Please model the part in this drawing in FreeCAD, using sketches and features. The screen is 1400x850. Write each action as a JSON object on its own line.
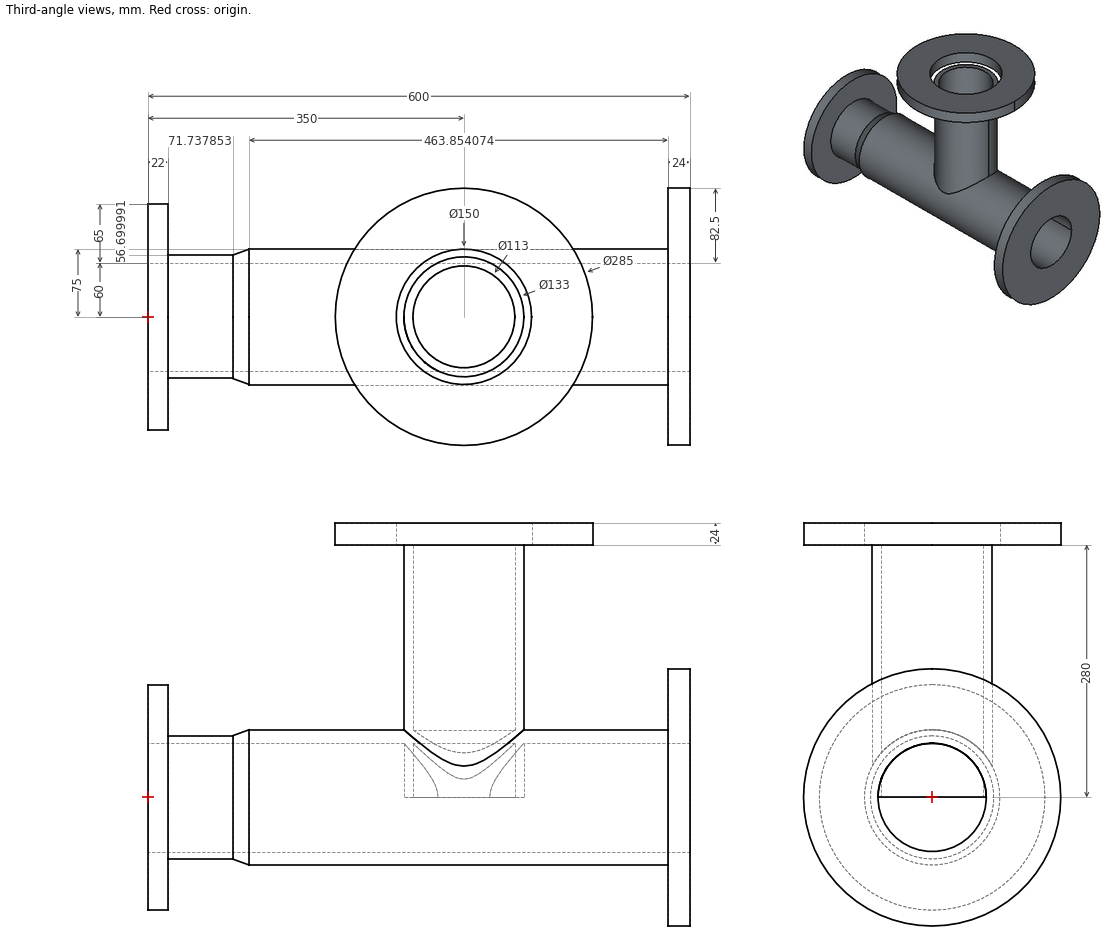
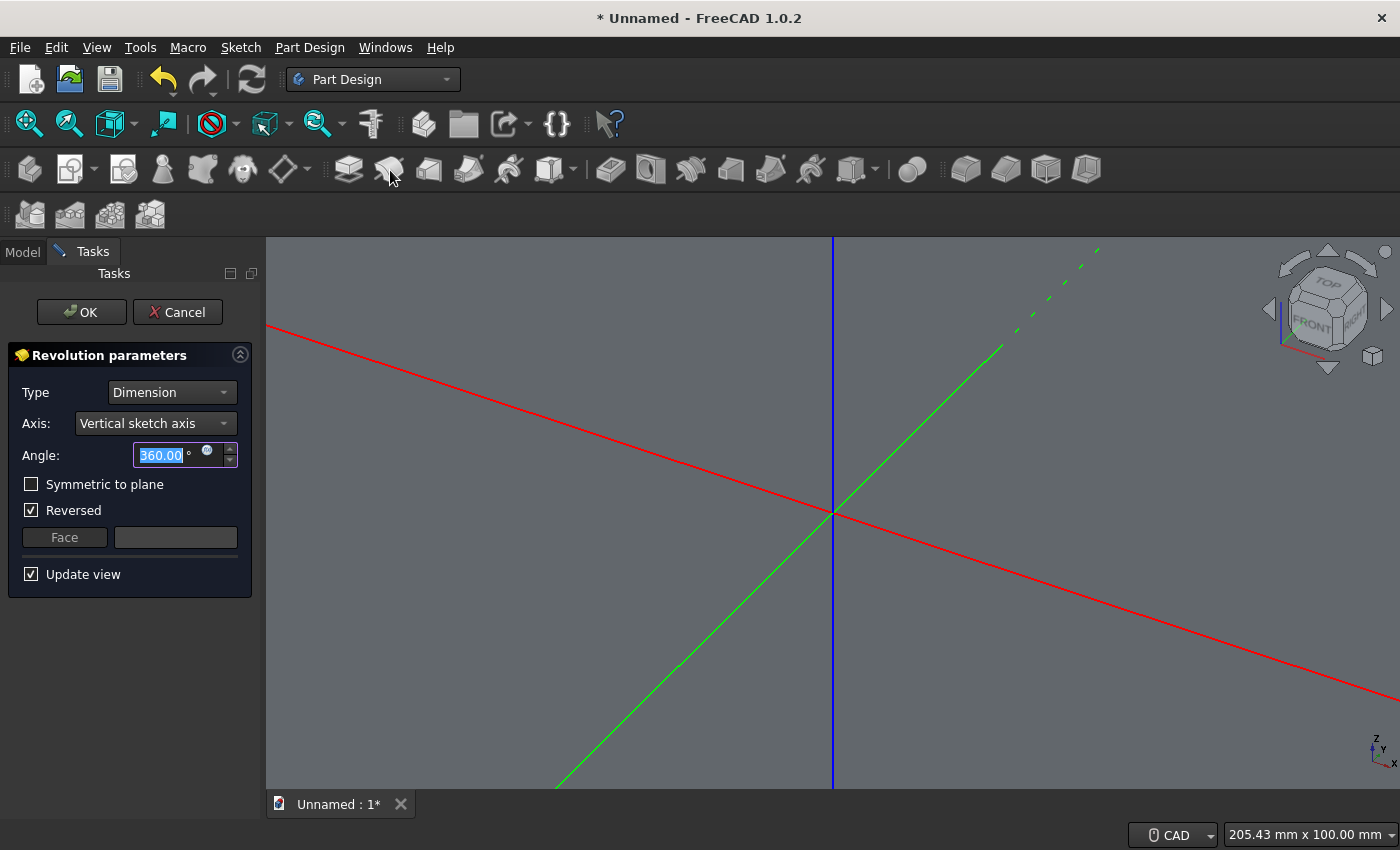
{"action": "left_click", "coordinate": [156, 424]}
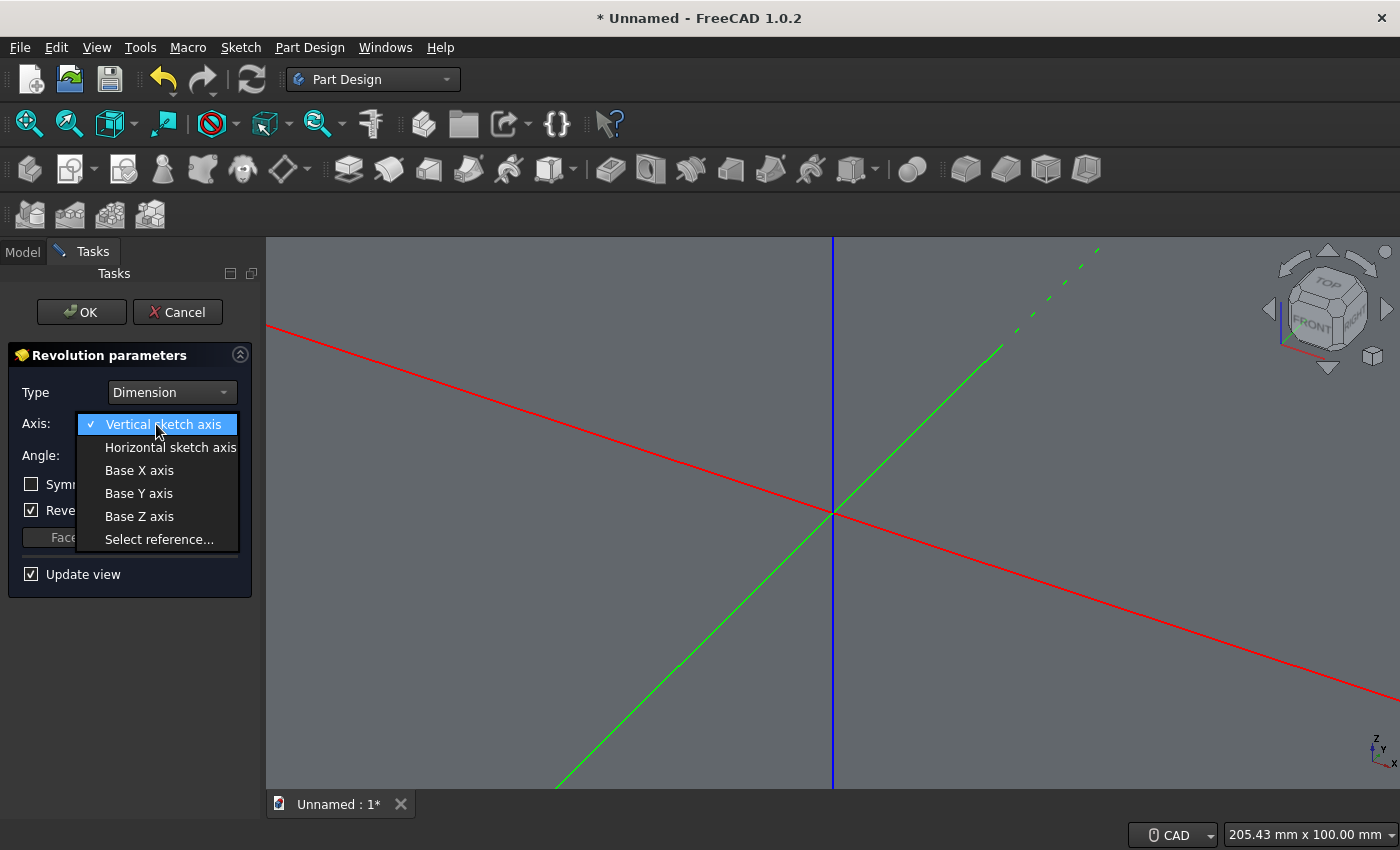
{"action": "left_click", "coordinate": [156, 448]}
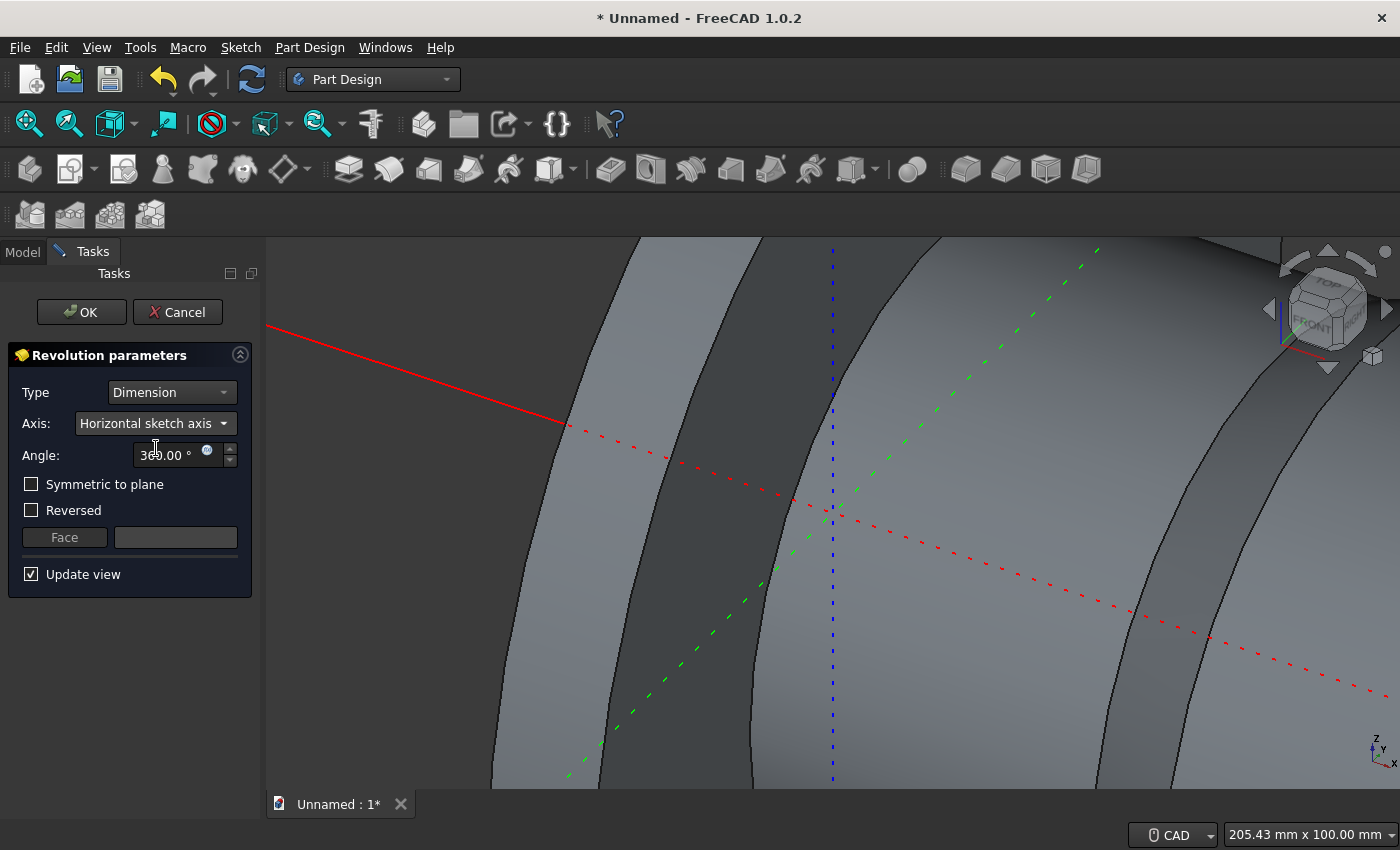
{"action": "left_click", "coordinate": [82, 312]}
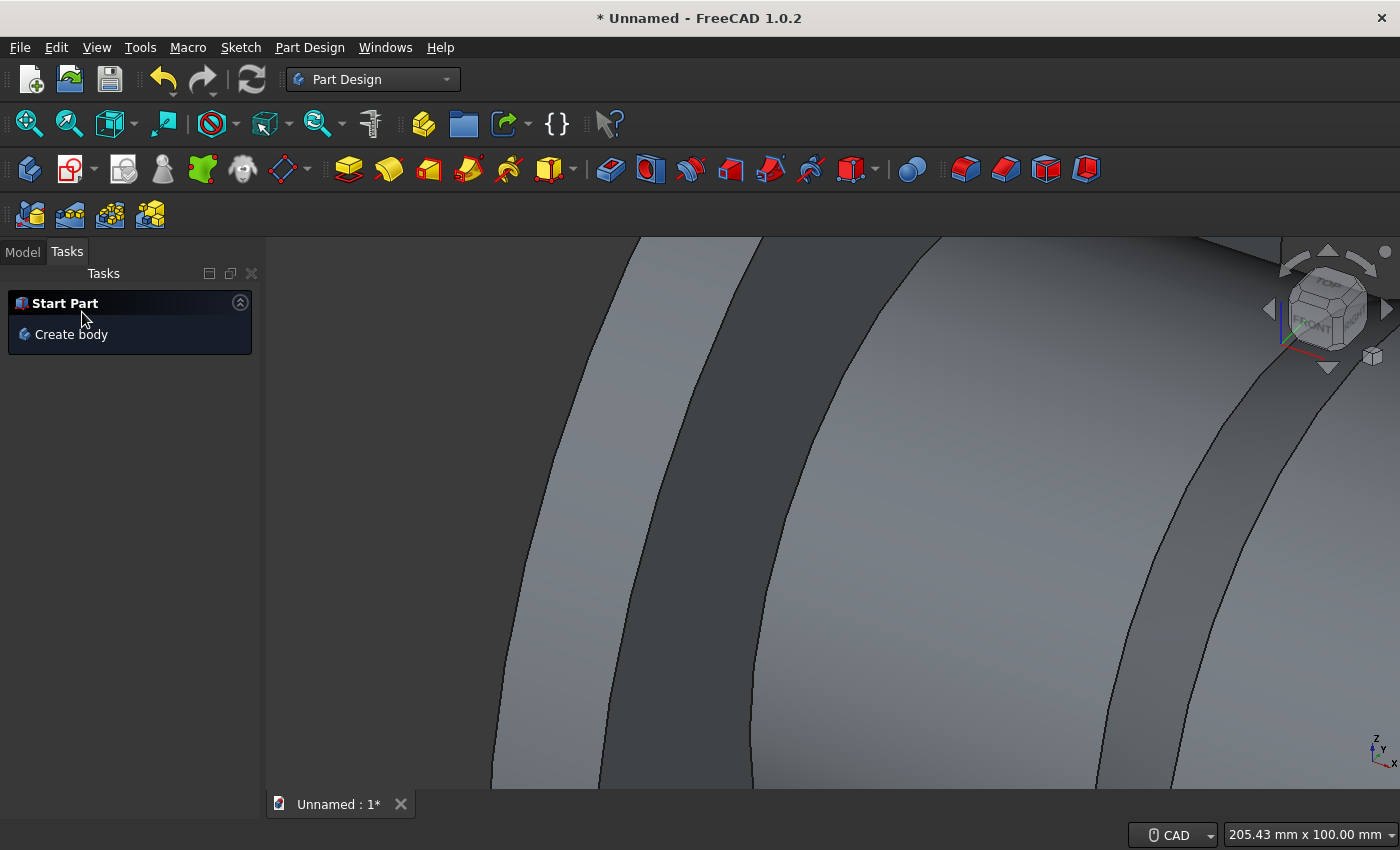
{"action": "key", "text": "v f"}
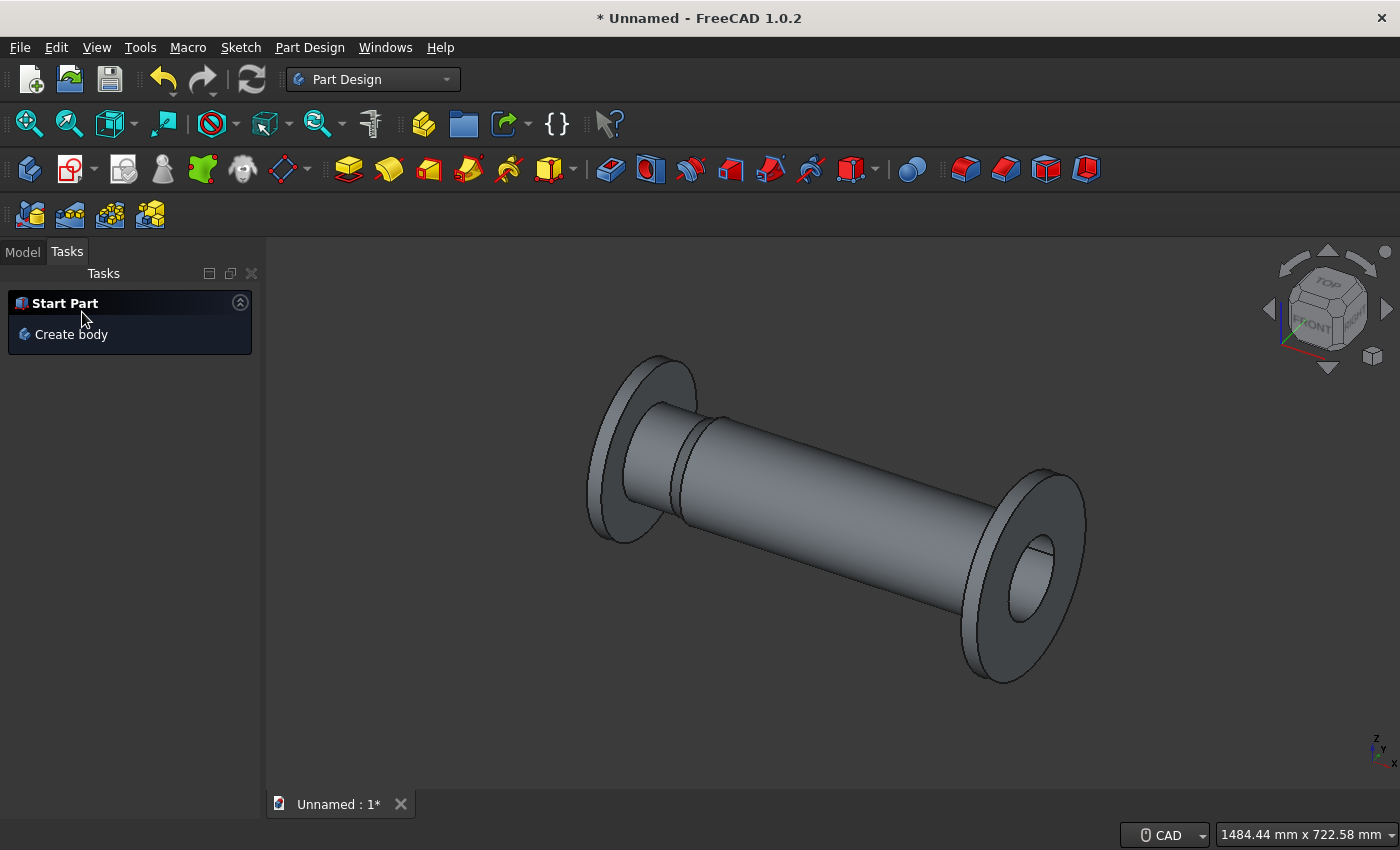
{"action": "left_click", "coordinate": [70, 170]}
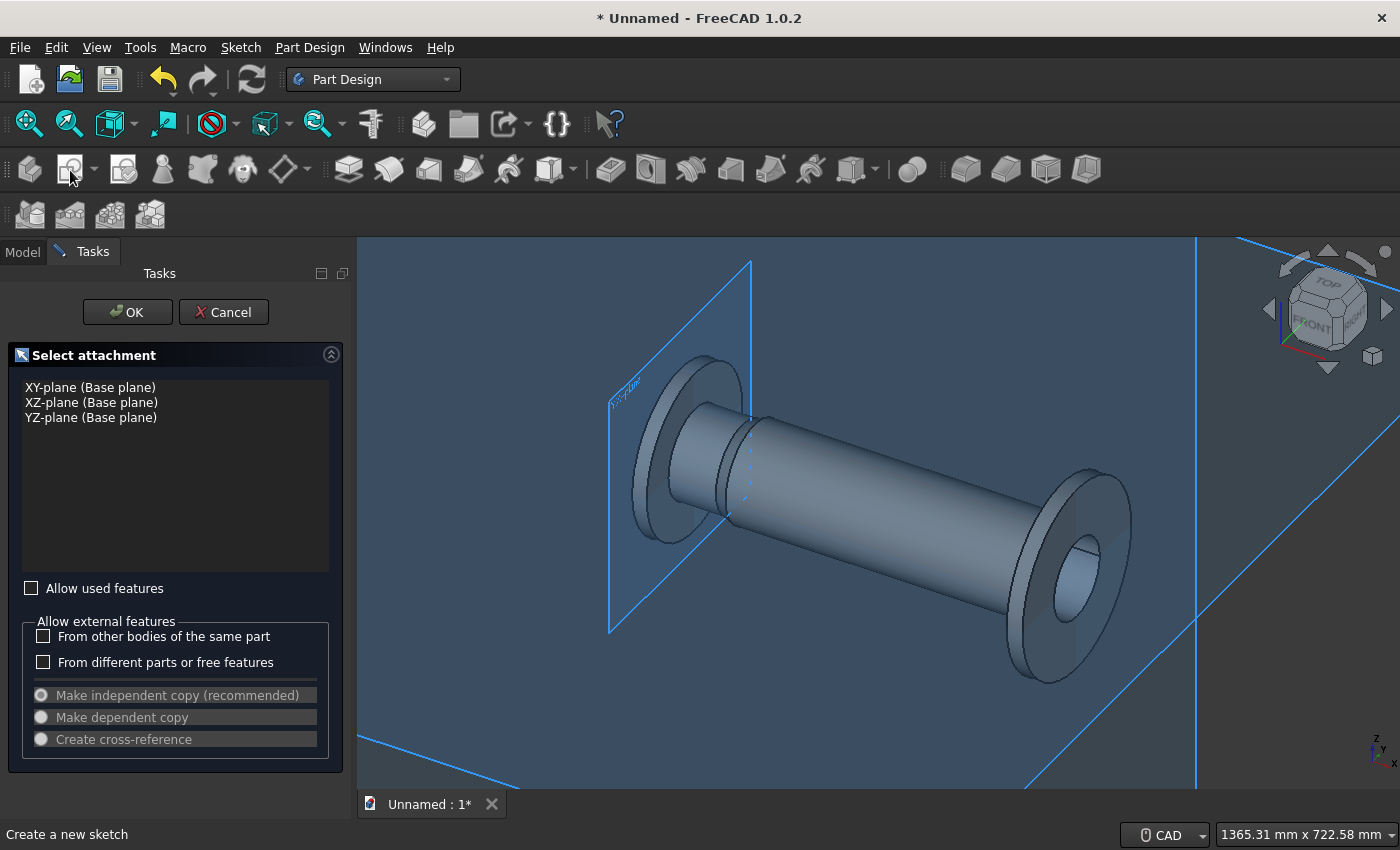
{"action": "left_click", "coordinate": [82, 388]}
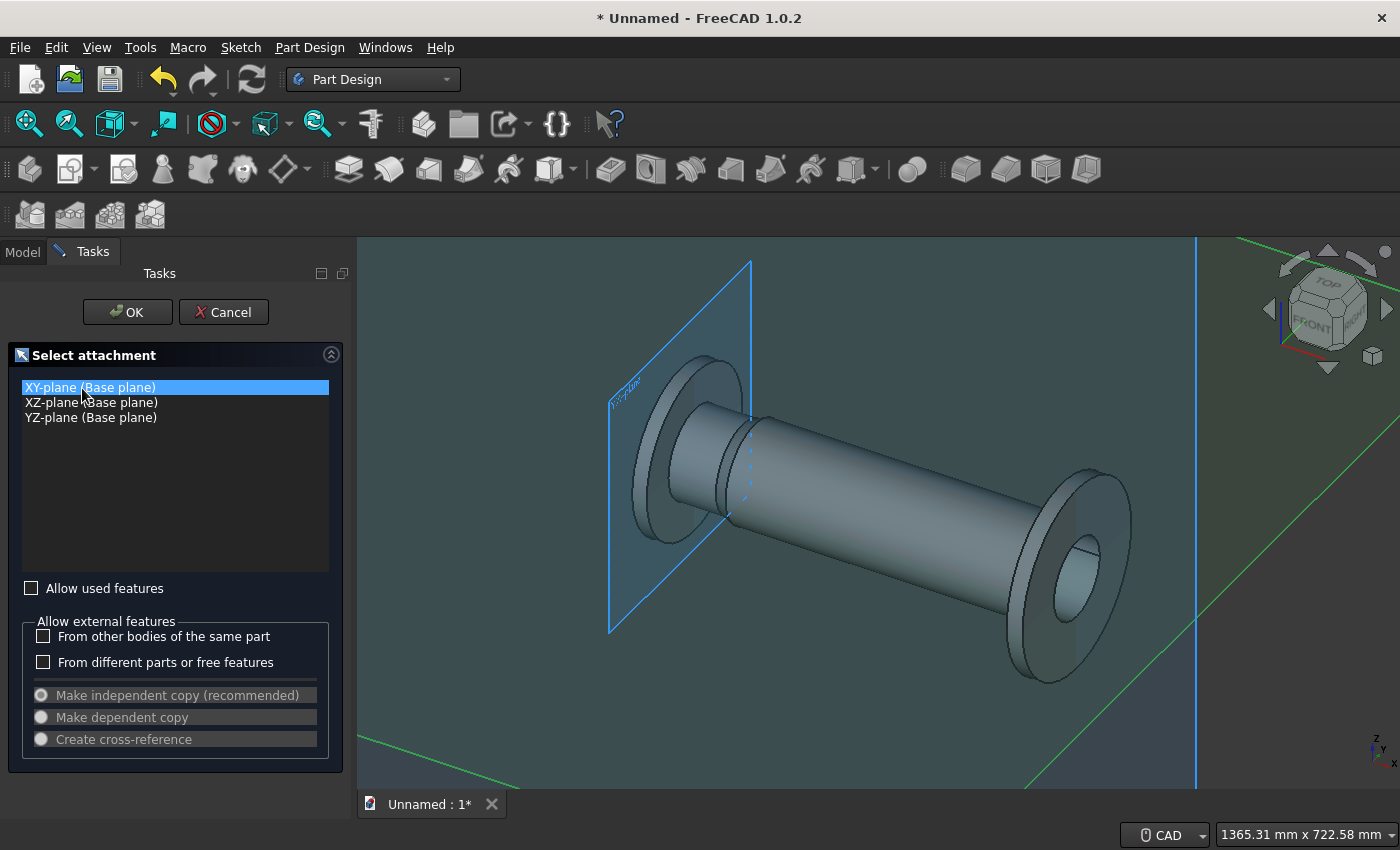
{"action": "left_click", "coordinate": [128, 312]}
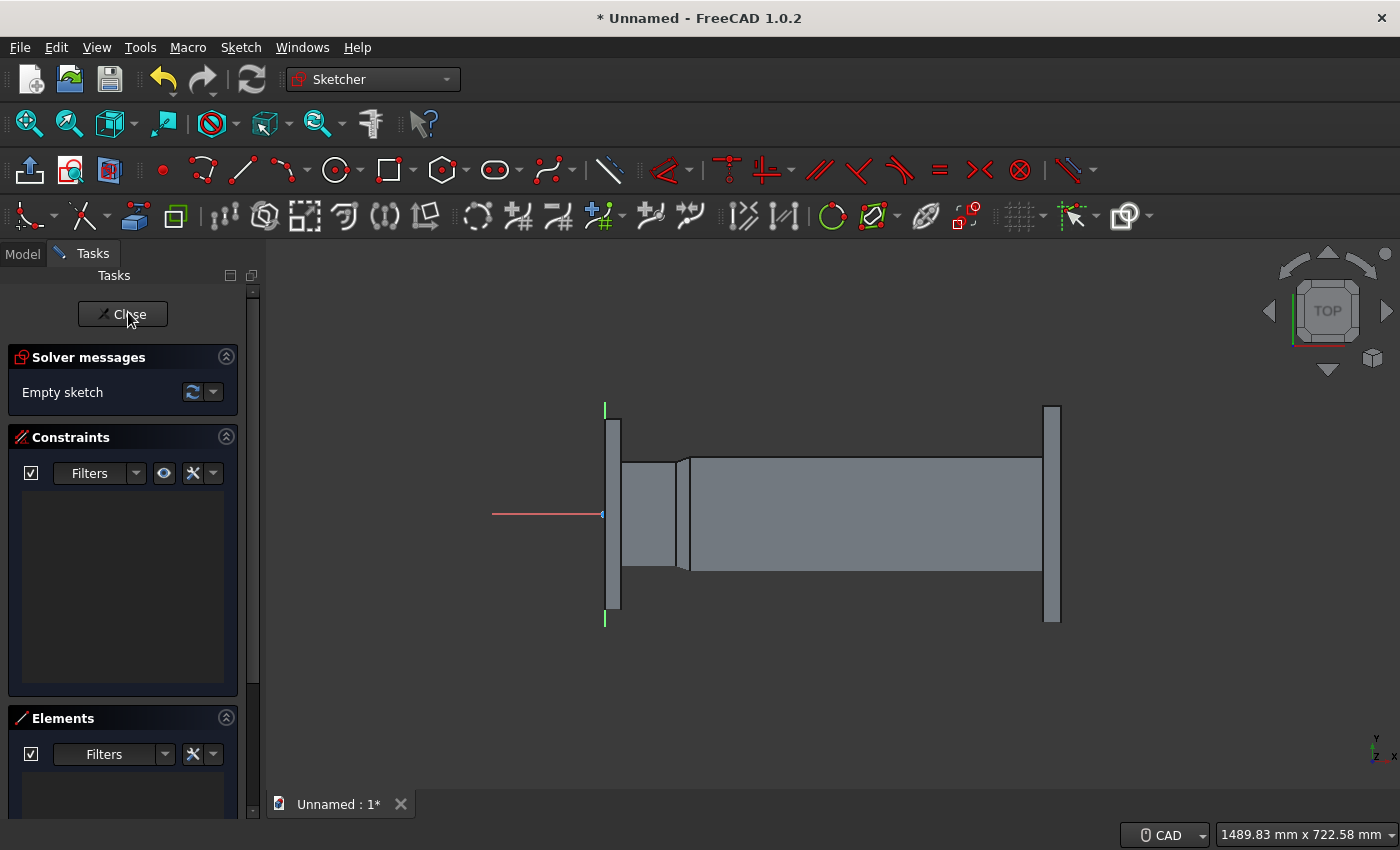
{"action": "key", "text": "q s"}